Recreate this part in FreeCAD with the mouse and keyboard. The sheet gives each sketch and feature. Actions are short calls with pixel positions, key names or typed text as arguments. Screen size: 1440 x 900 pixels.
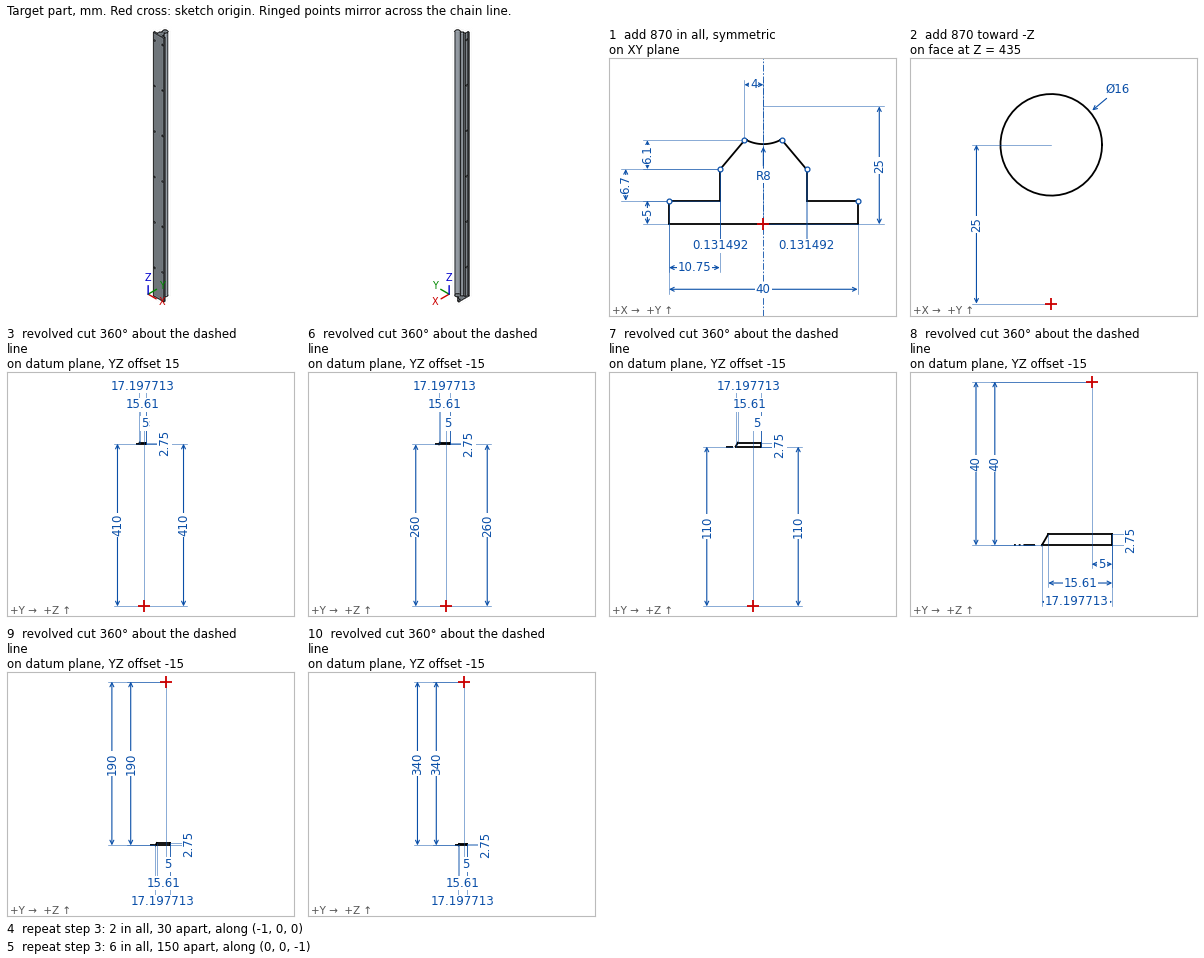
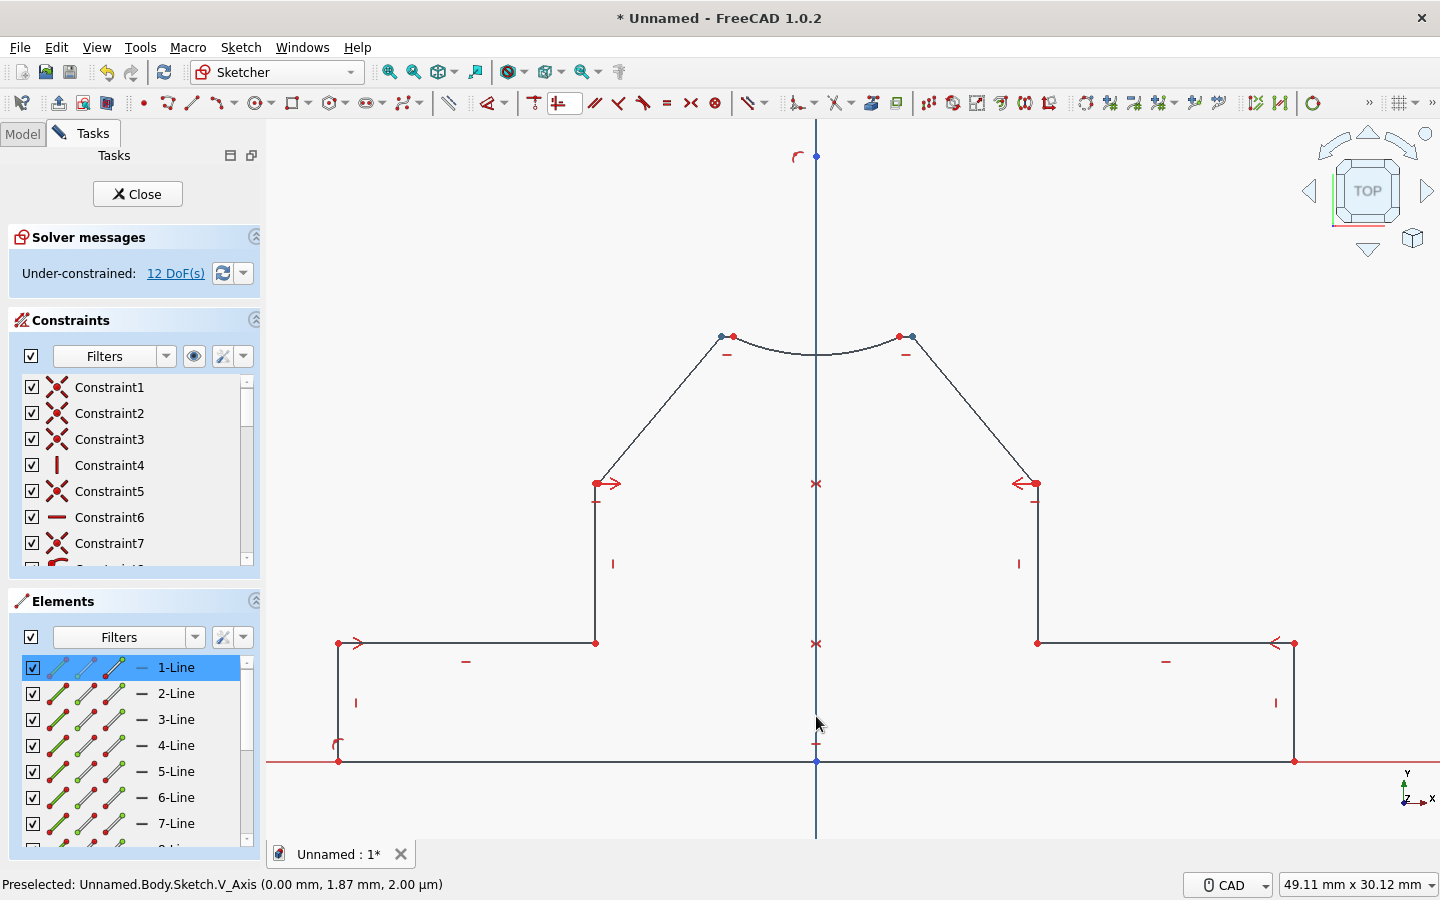
key(s)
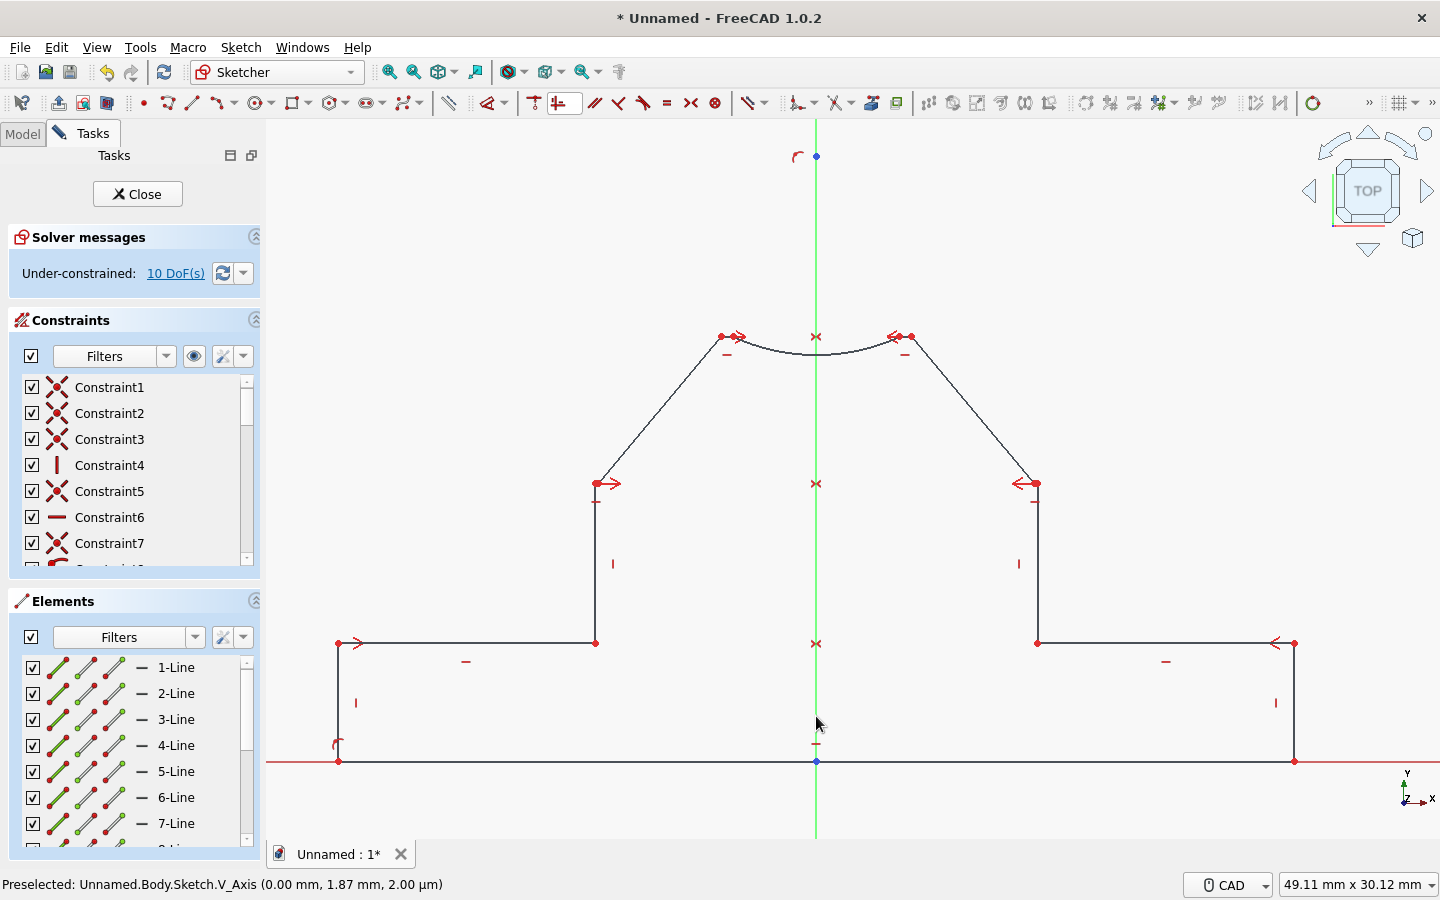
click(488, 104)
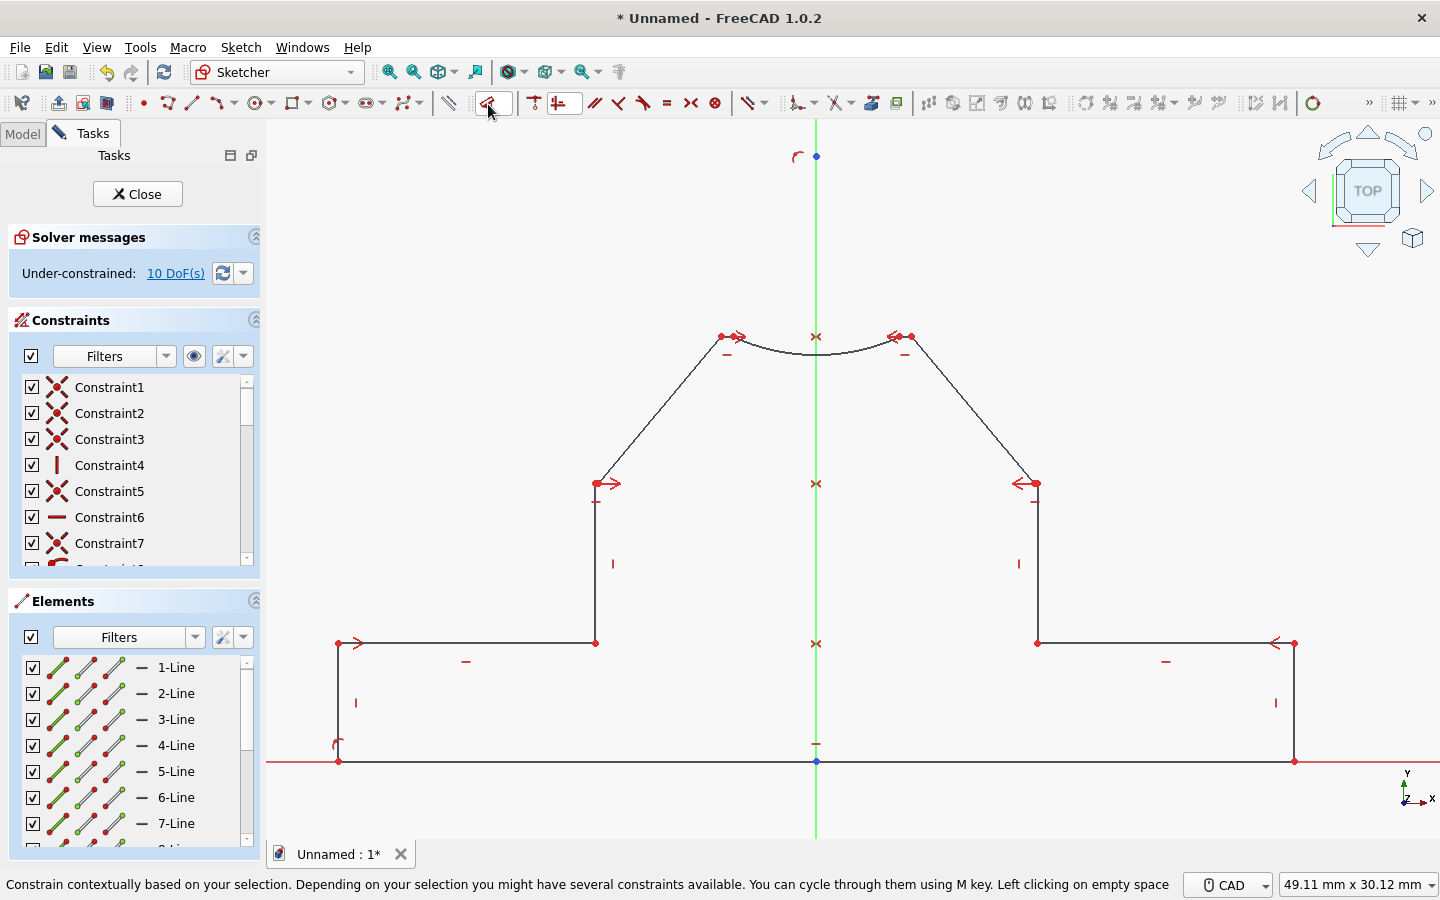
click(782, 352)
click(776, 384)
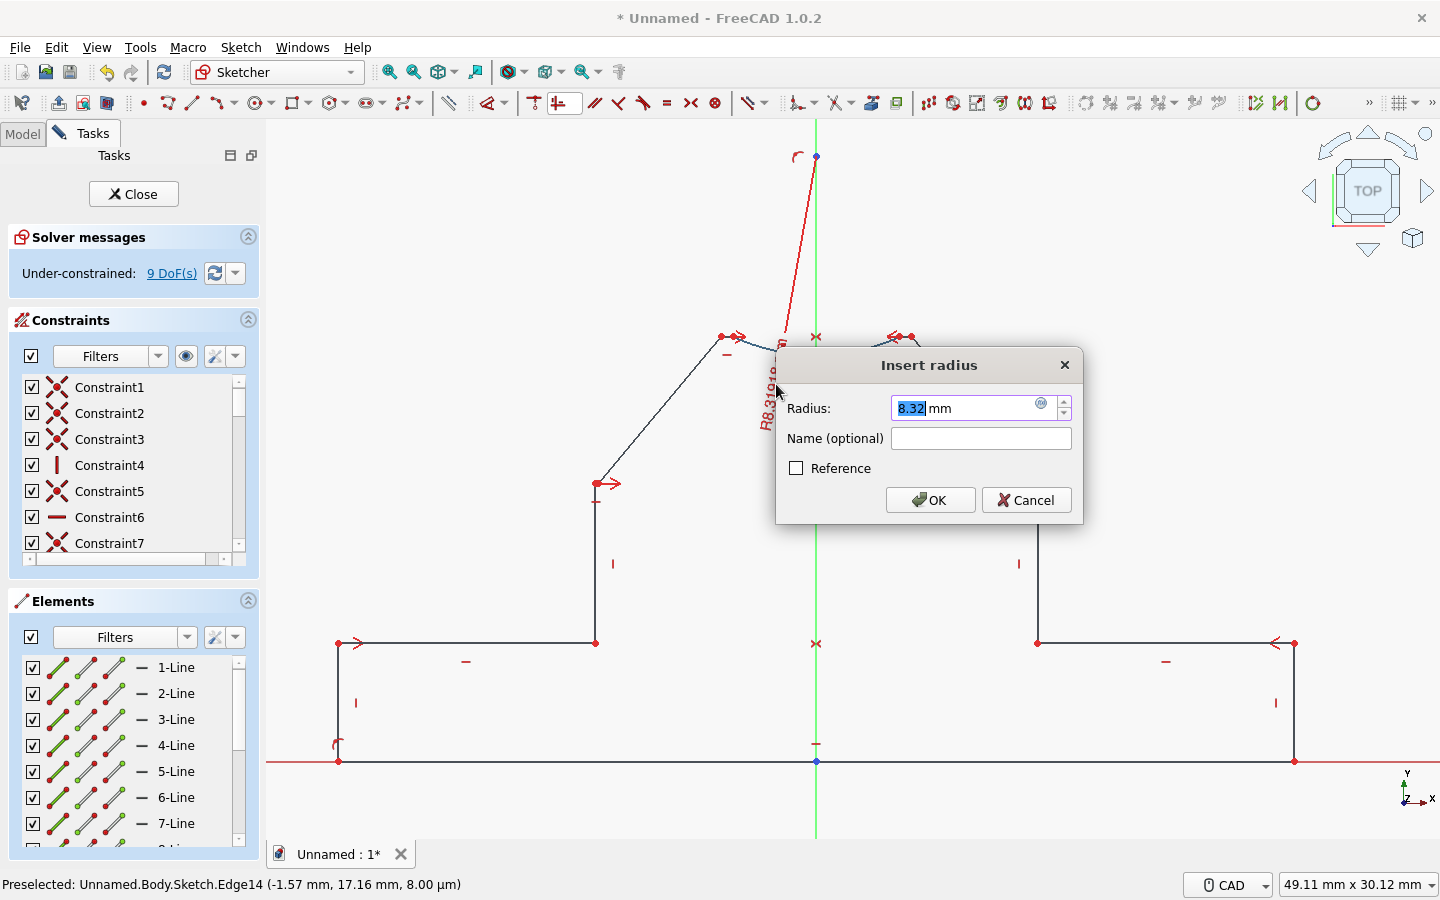
text(8)
key(Return)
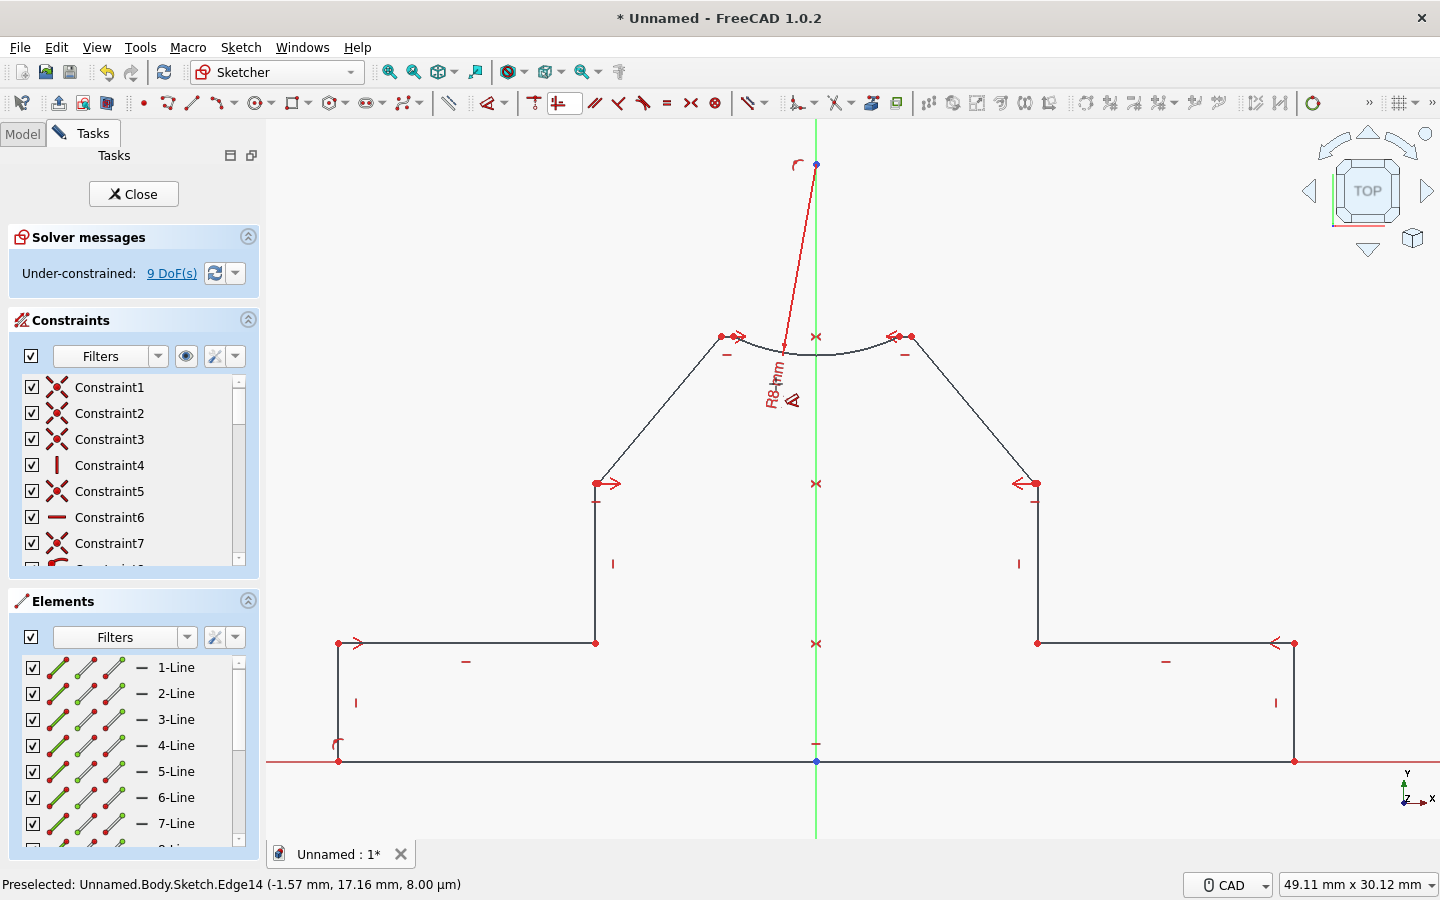
click(338, 679)
click(304, 702)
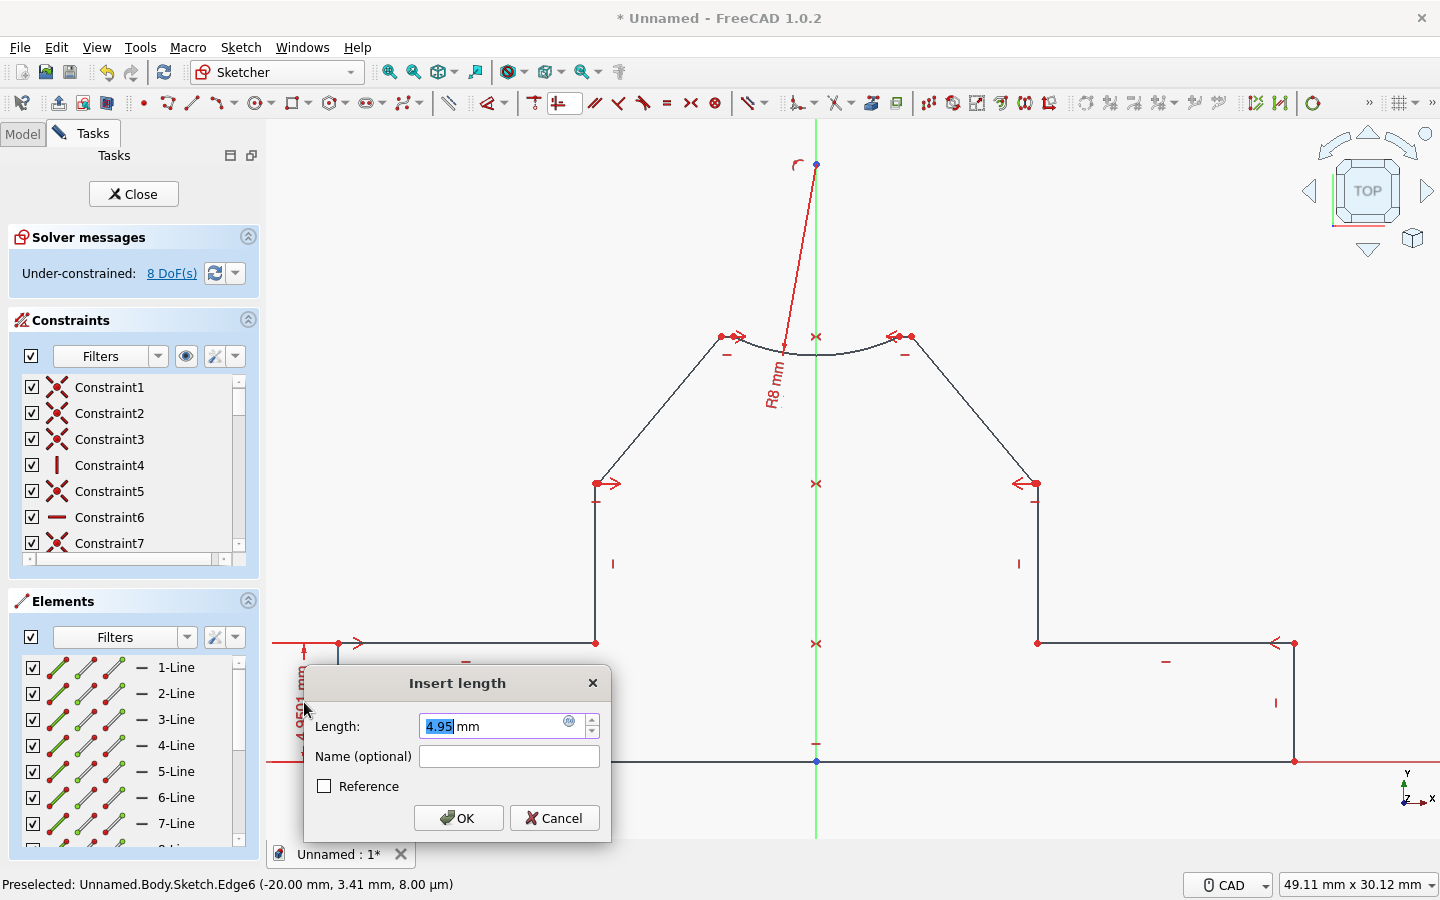
text(5)
key(Return)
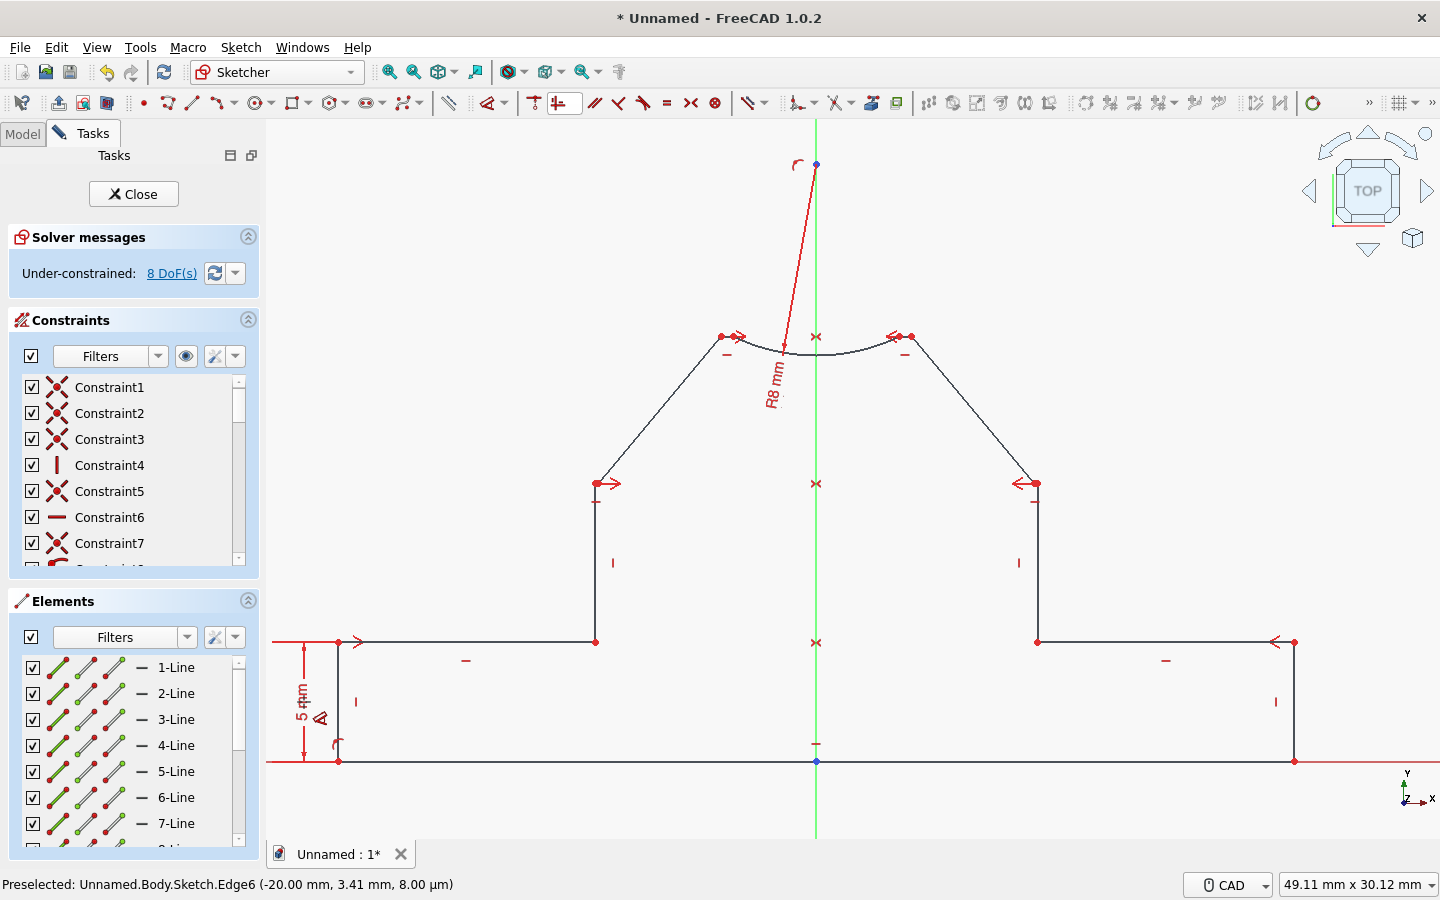
click(625, 762)
click(591, 796)